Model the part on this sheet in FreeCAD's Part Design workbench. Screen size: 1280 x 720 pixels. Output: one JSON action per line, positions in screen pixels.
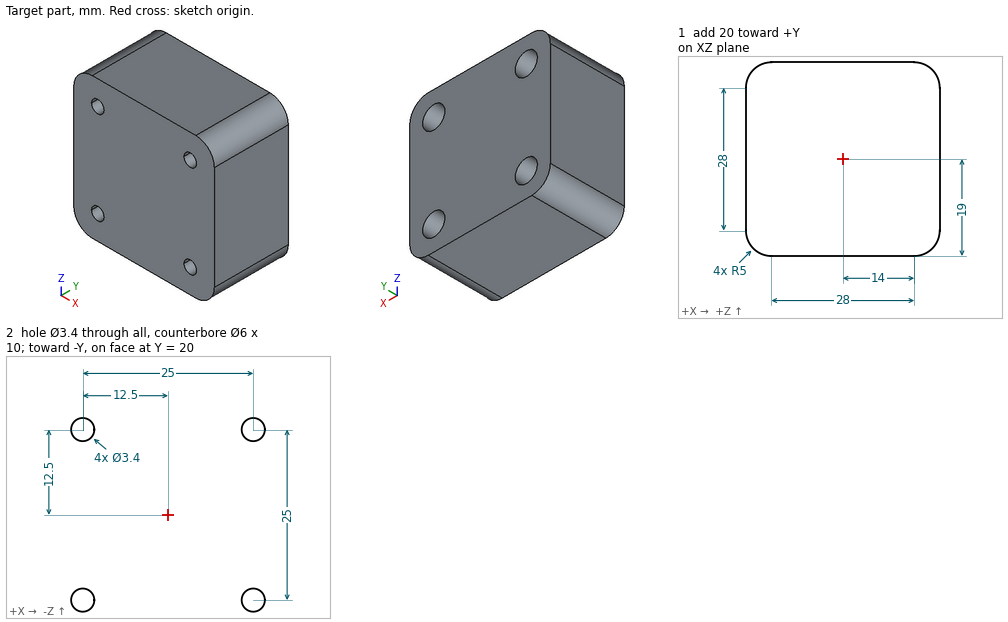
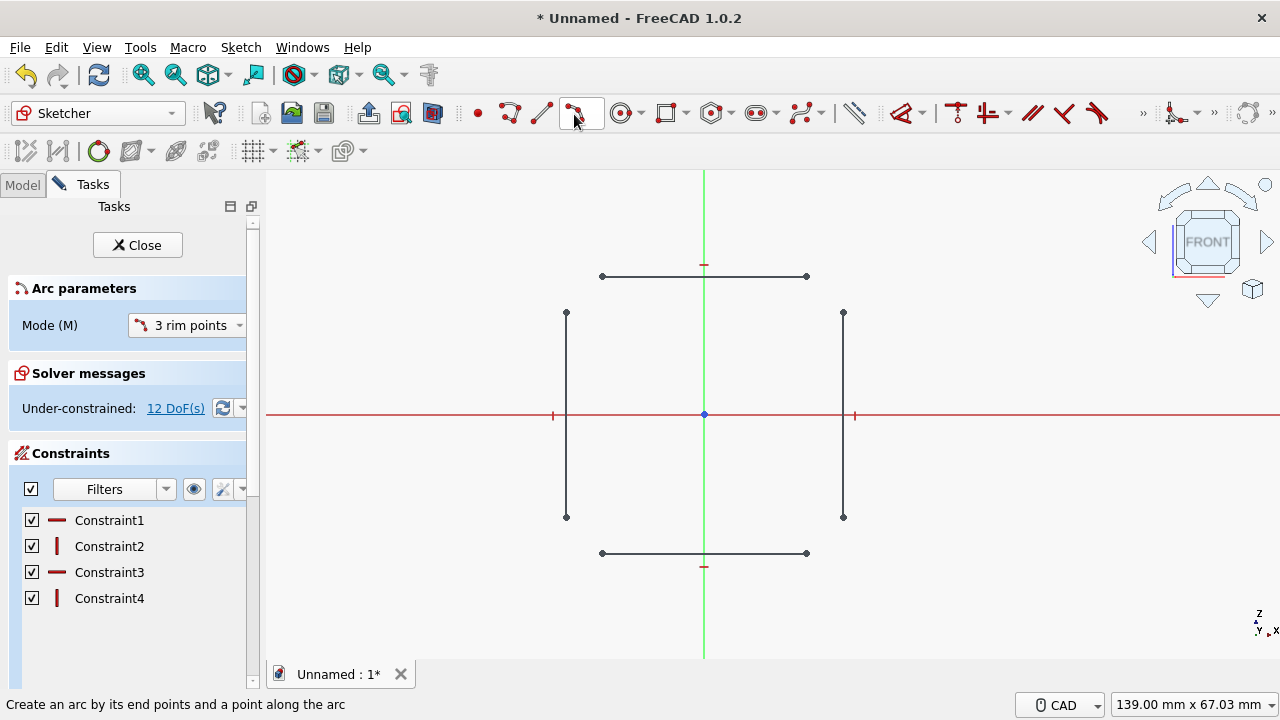
{"action": "left_click", "coordinate": [602, 554]}
{"action": "left_click", "coordinate": [566, 518]}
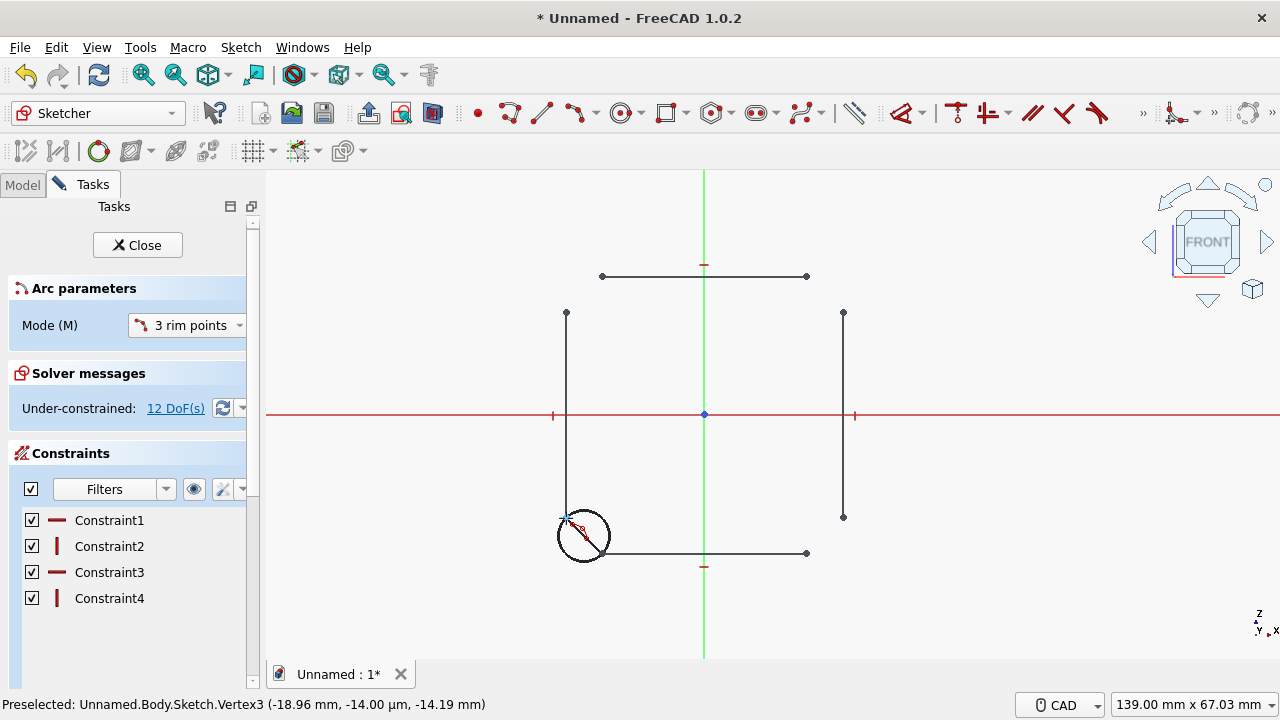
{"action": "scroll", "coordinate": [576, 542], "scroll_direction": "up", "scroll_amount": 2}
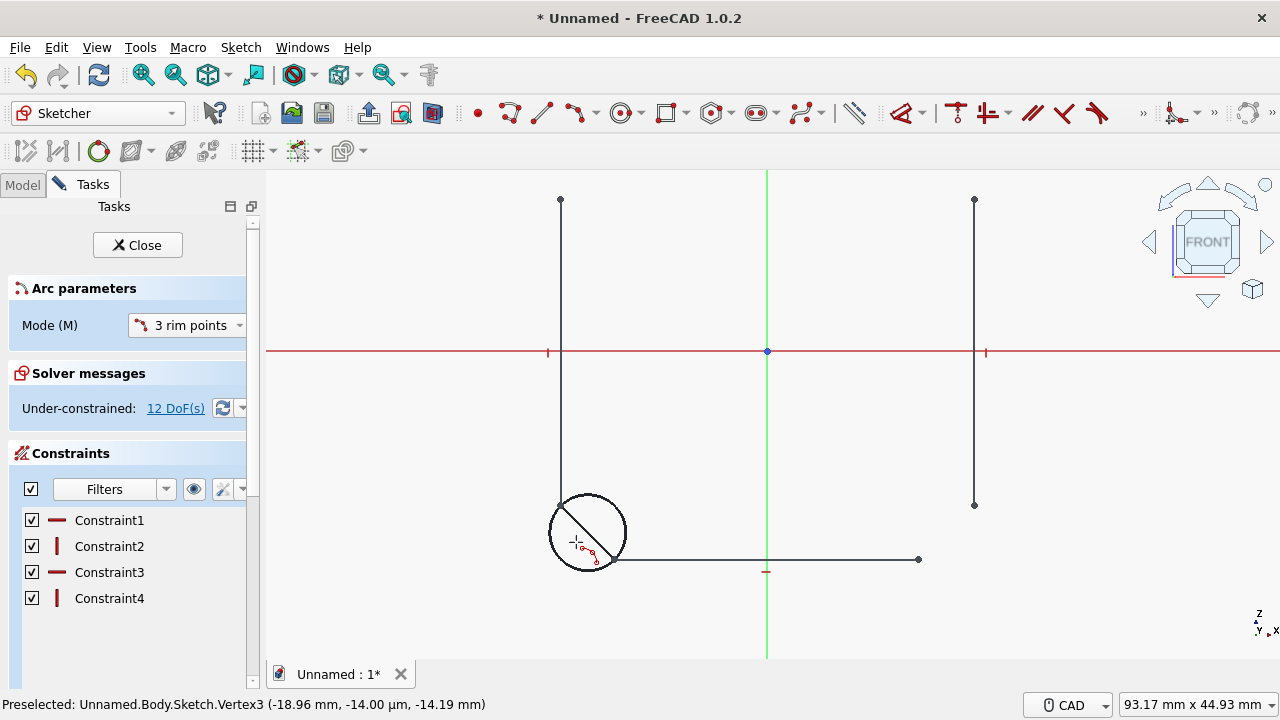
{"action": "left_click", "coordinate": [576, 542]}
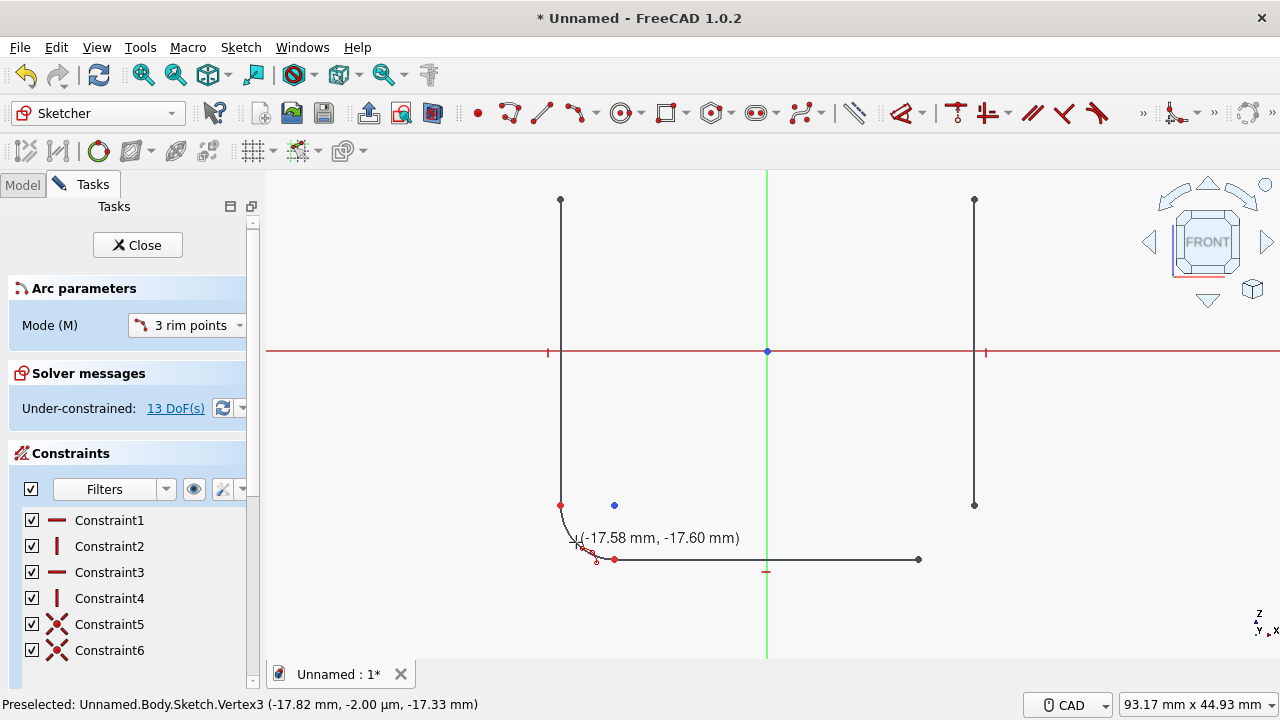
{"action": "left_click", "coordinate": [561, 200]}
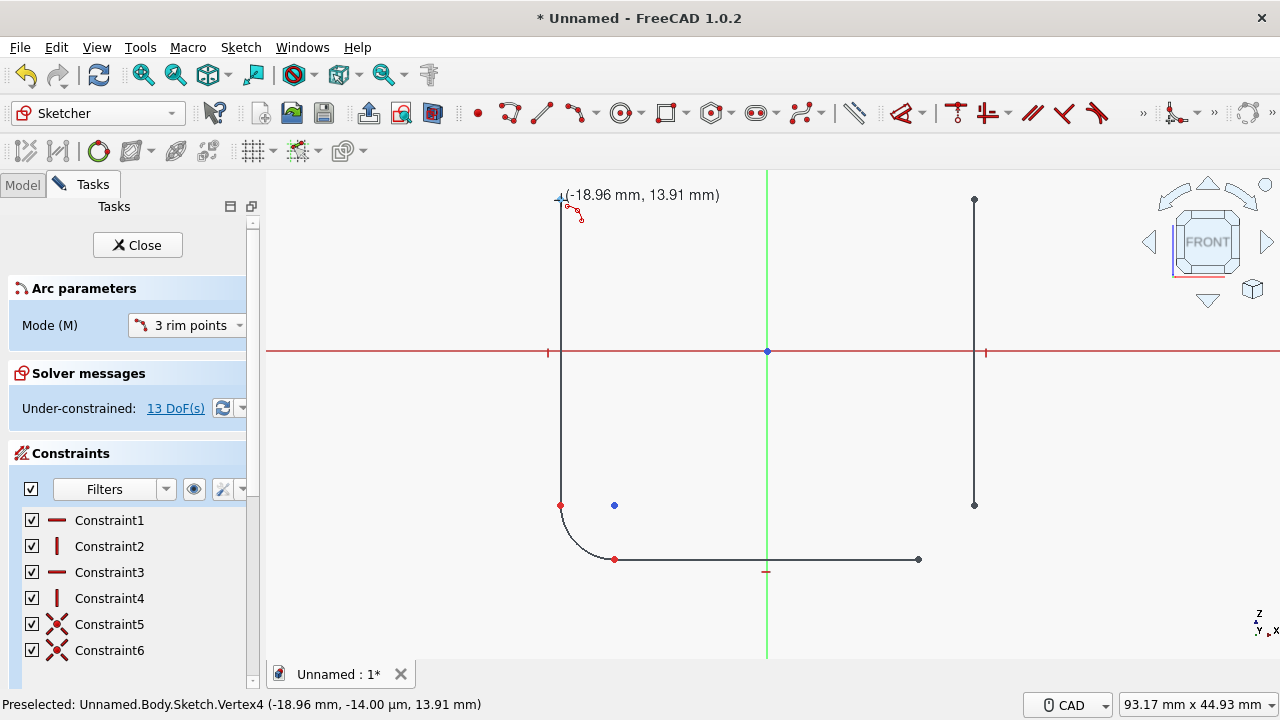
{"action": "scroll", "coordinate": [577, 543], "scroll_direction": "down", "scroll_amount": 2}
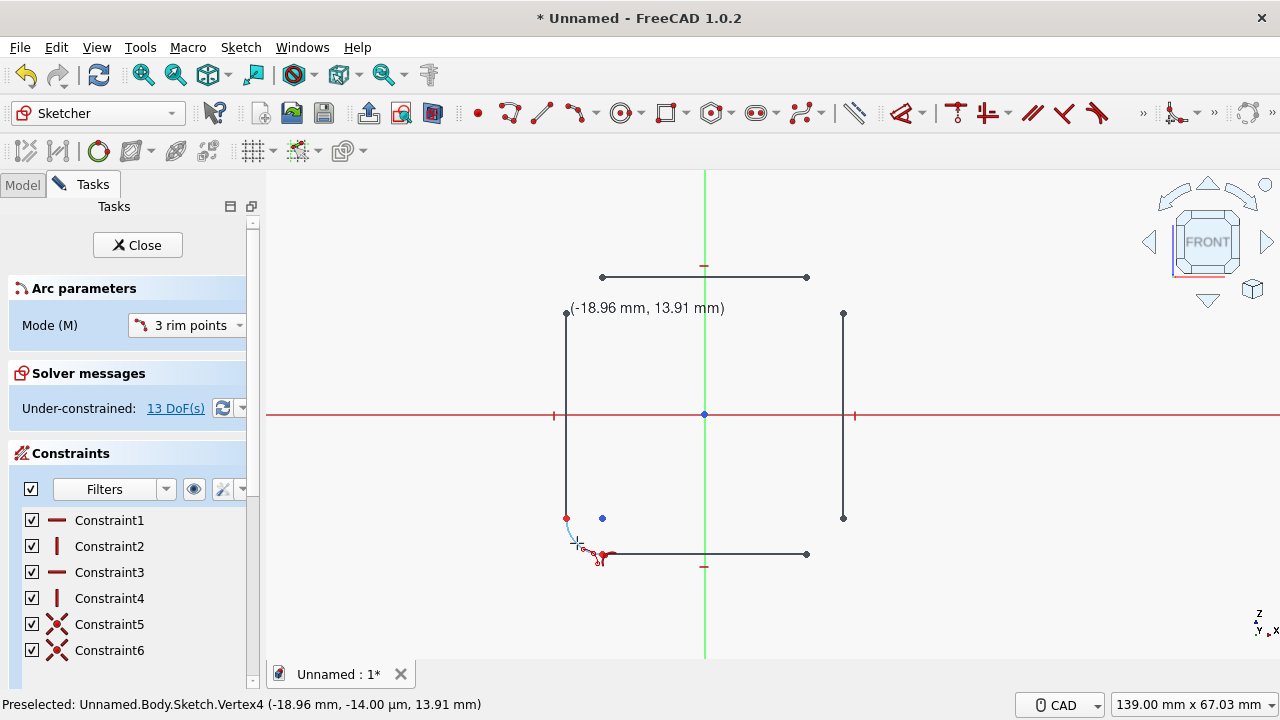
{"action": "left_click", "coordinate": [602, 277]}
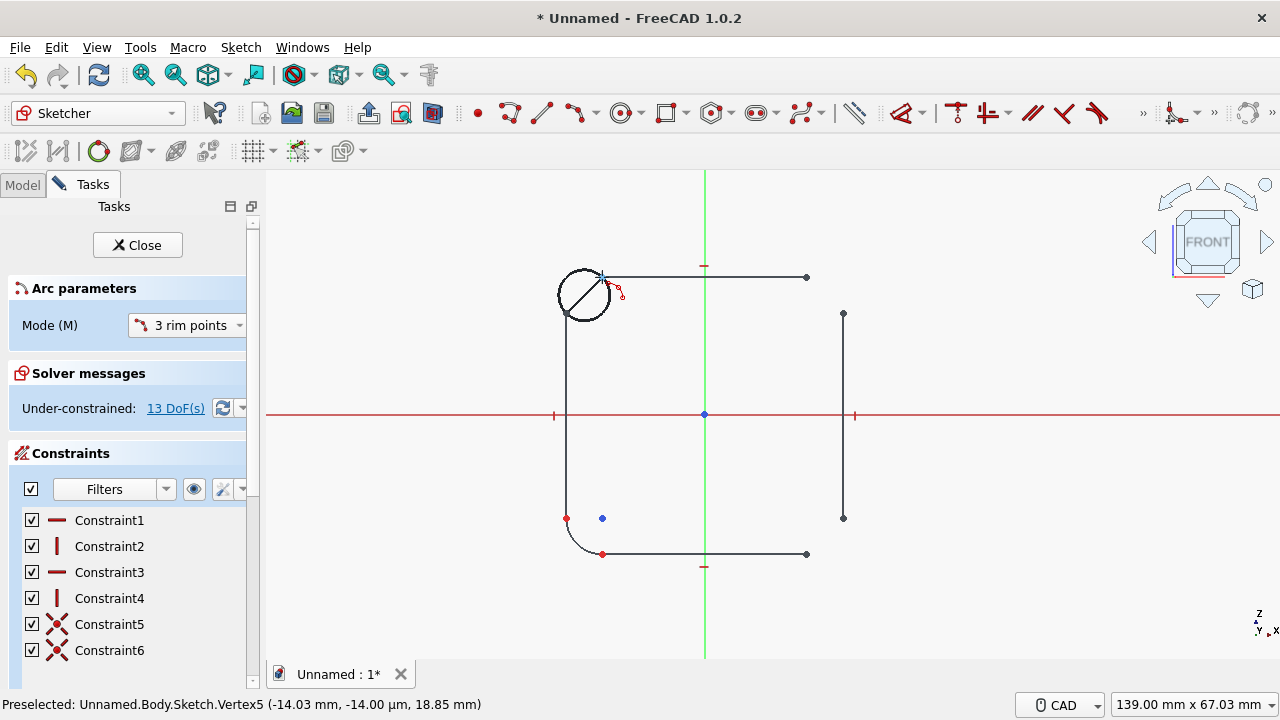
{"action": "scroll", "coordinate": [577, 287], "scroll_direction": "up", "scroll_amount": 2}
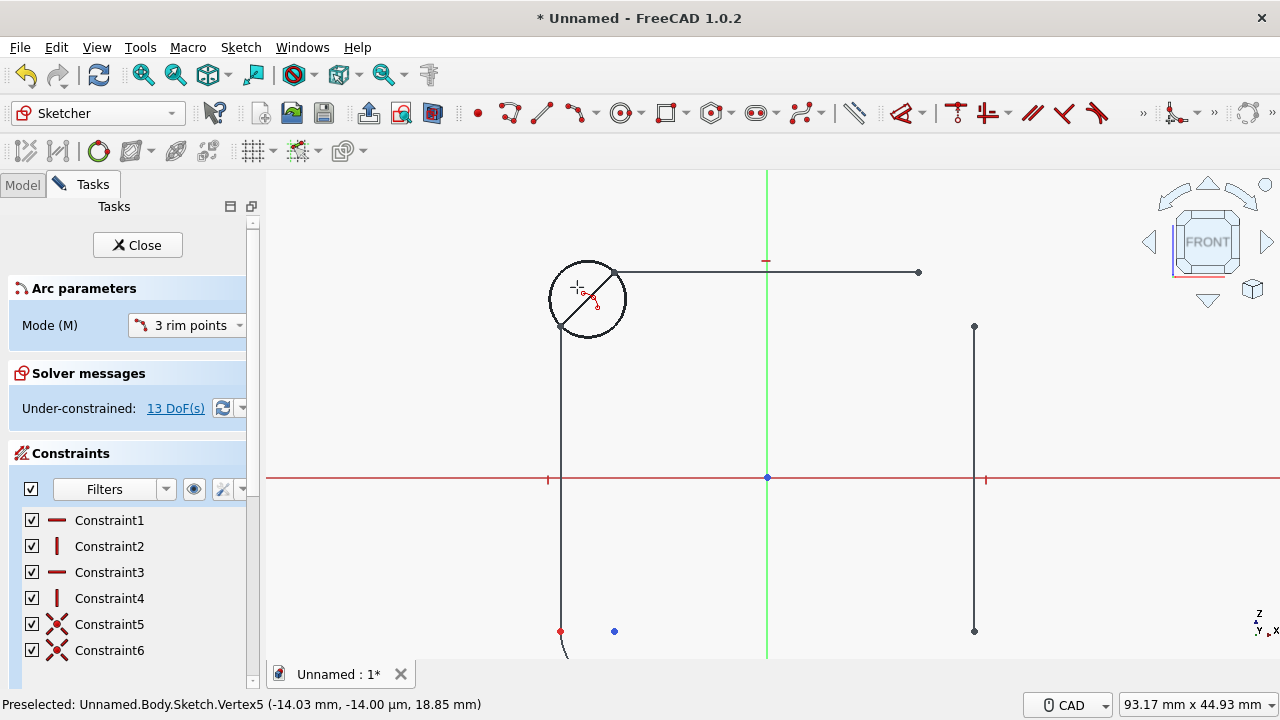
{"action": "left_click", "coordinate": [576, 287]}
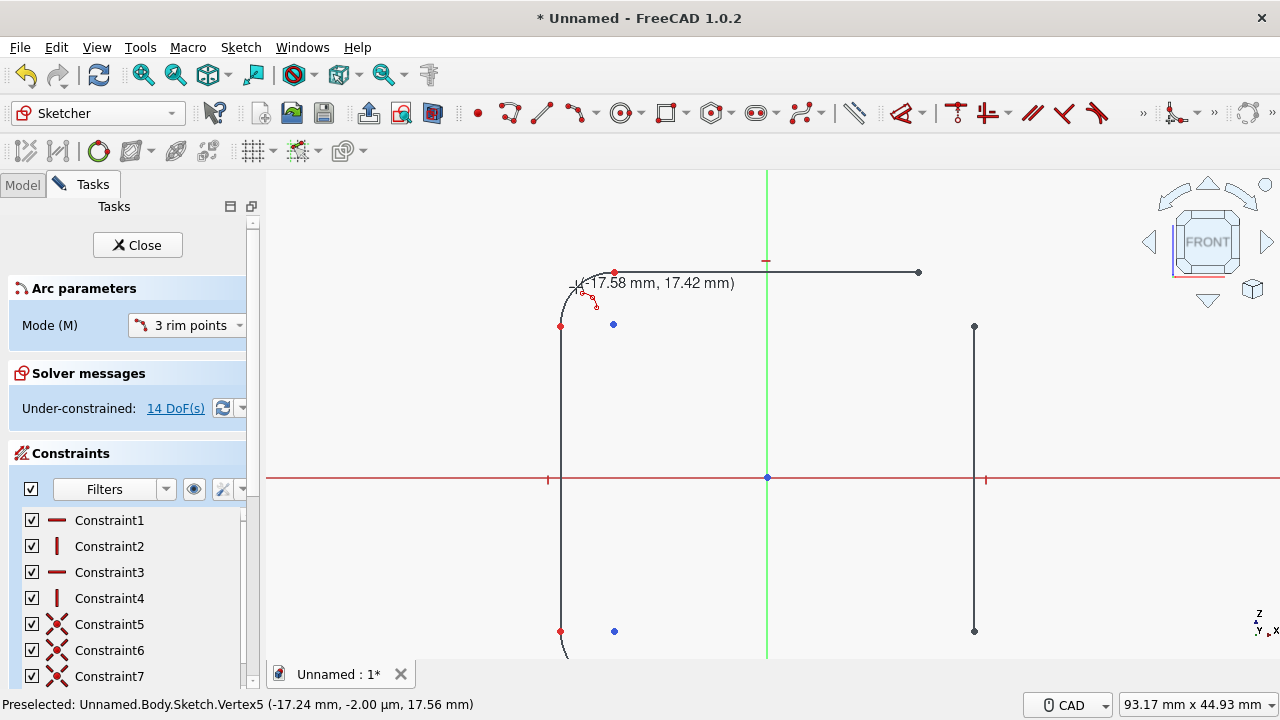
{"action": "left_click", "coordinate": [919, 272]}
{"action": "left_click", "coordinate": [974, 326]}
{"action": "left_click", "coordinate": [958, 287]}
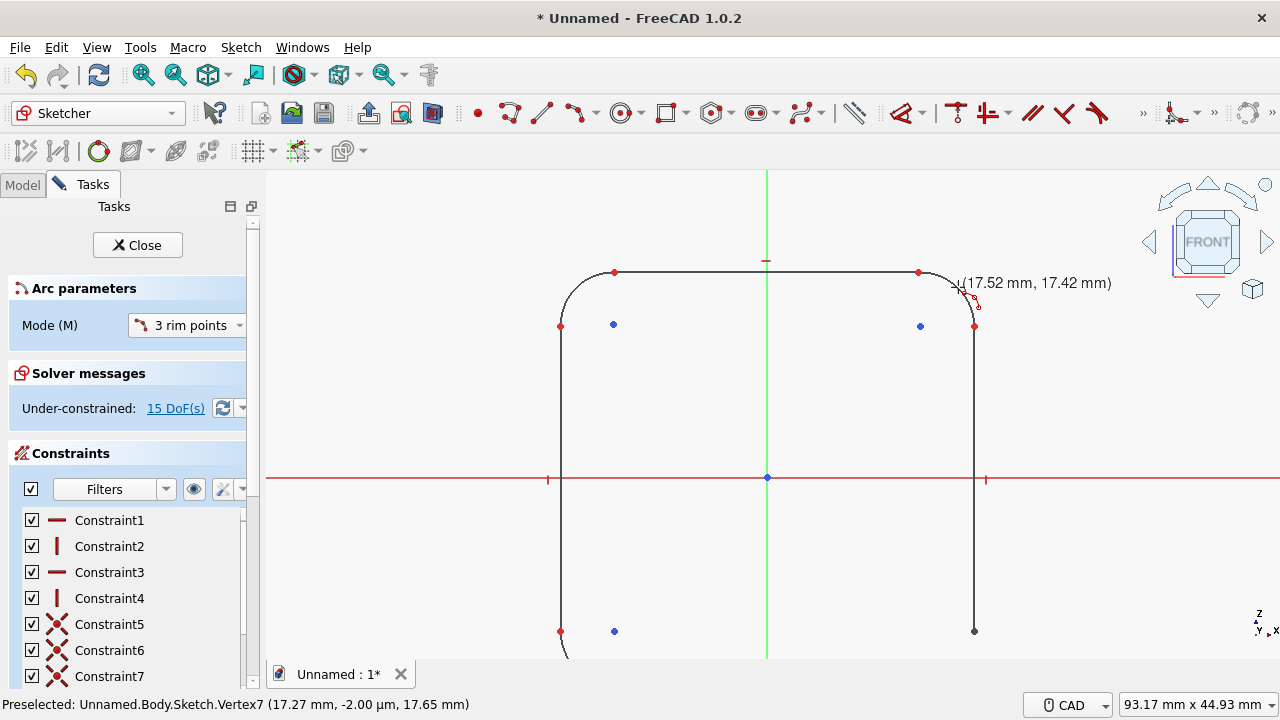
{"action": "left_click", "coordinate": [974, 632]}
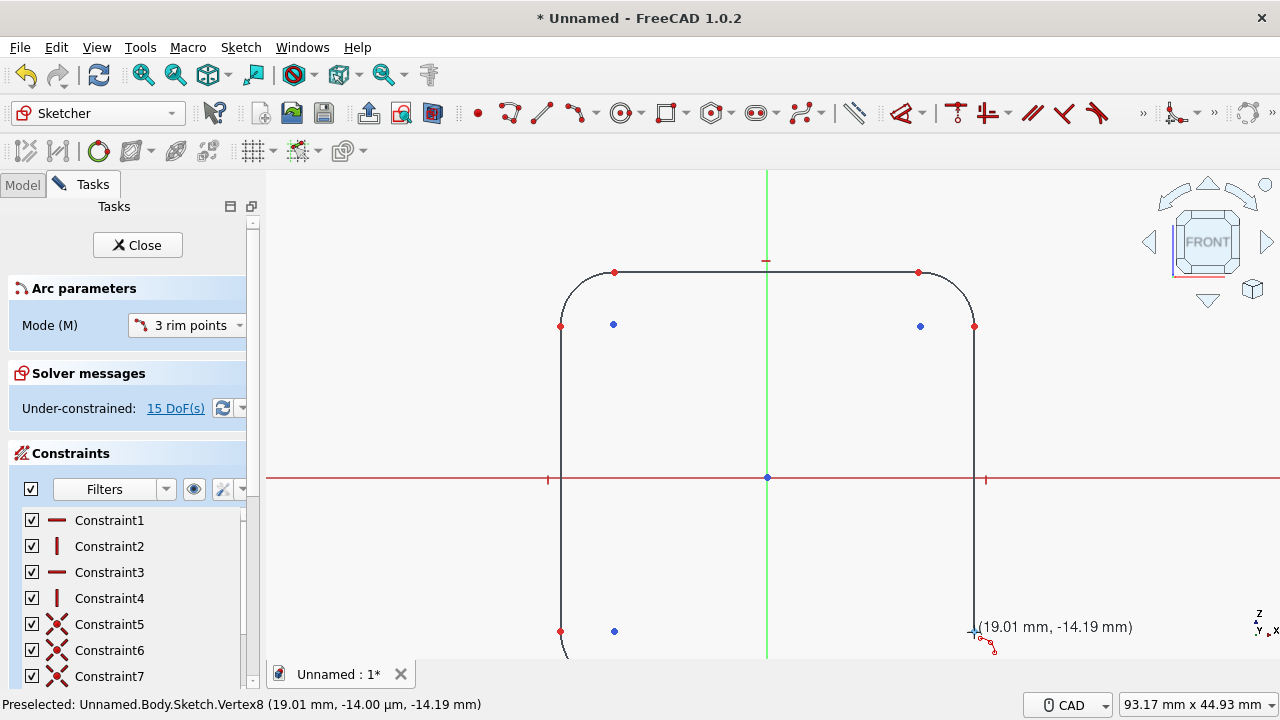
{"action": "scroll", "coordinate": [577, 286], "scroll_direction": "down", "scroll_amount": 2}